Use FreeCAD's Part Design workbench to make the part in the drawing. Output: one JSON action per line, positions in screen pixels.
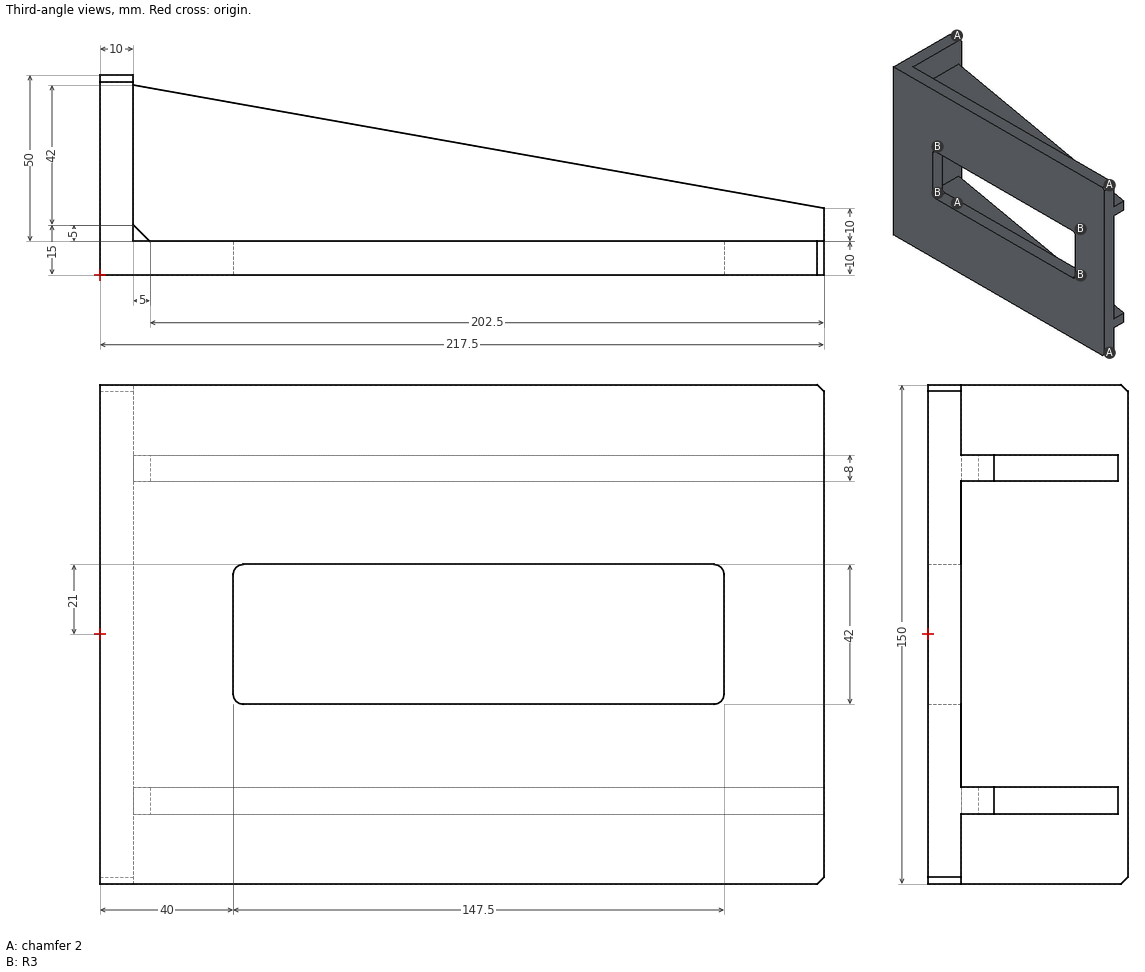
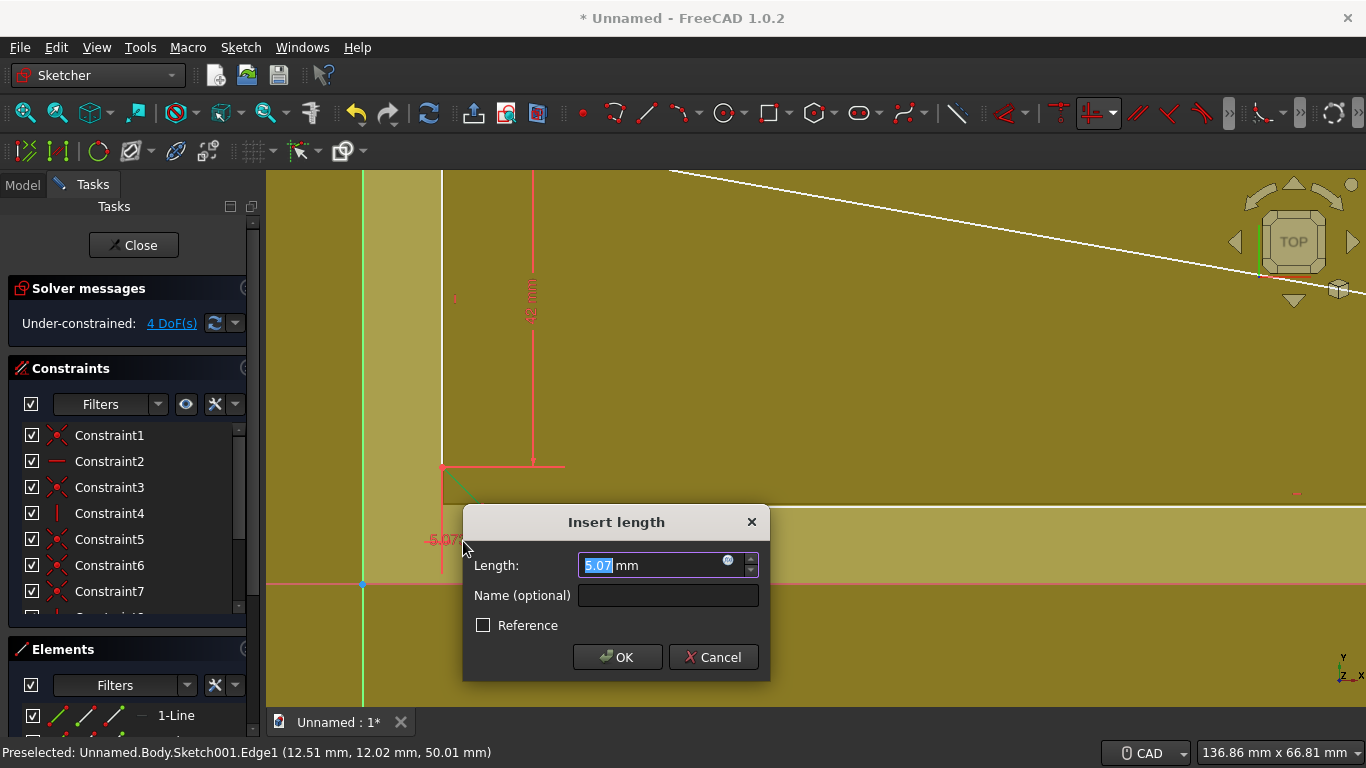
{"action": "type", "text": "5"}
{"action": "key", "text": "Return"}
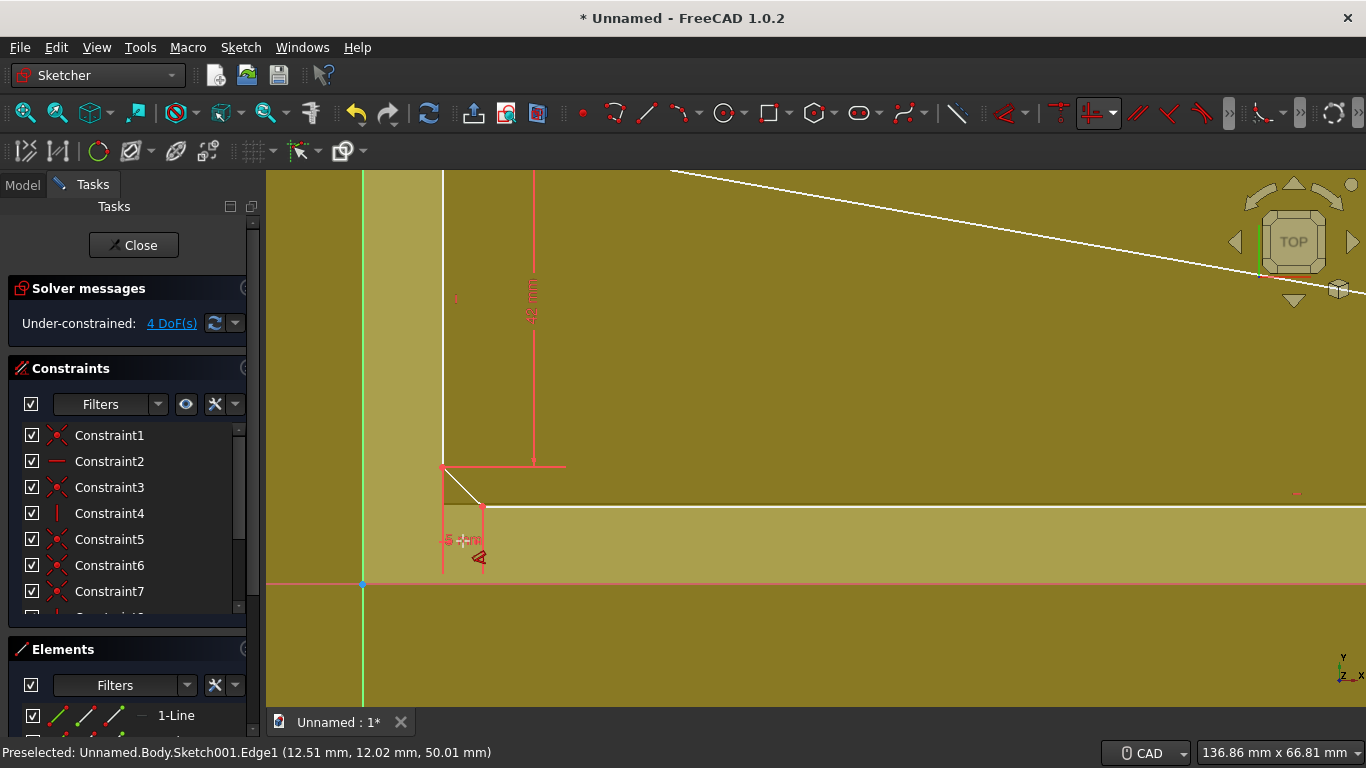
{"action": "left_click", "coordinate": [455, 479]}
{"action": "left_click", "coordinate": [409, 487]}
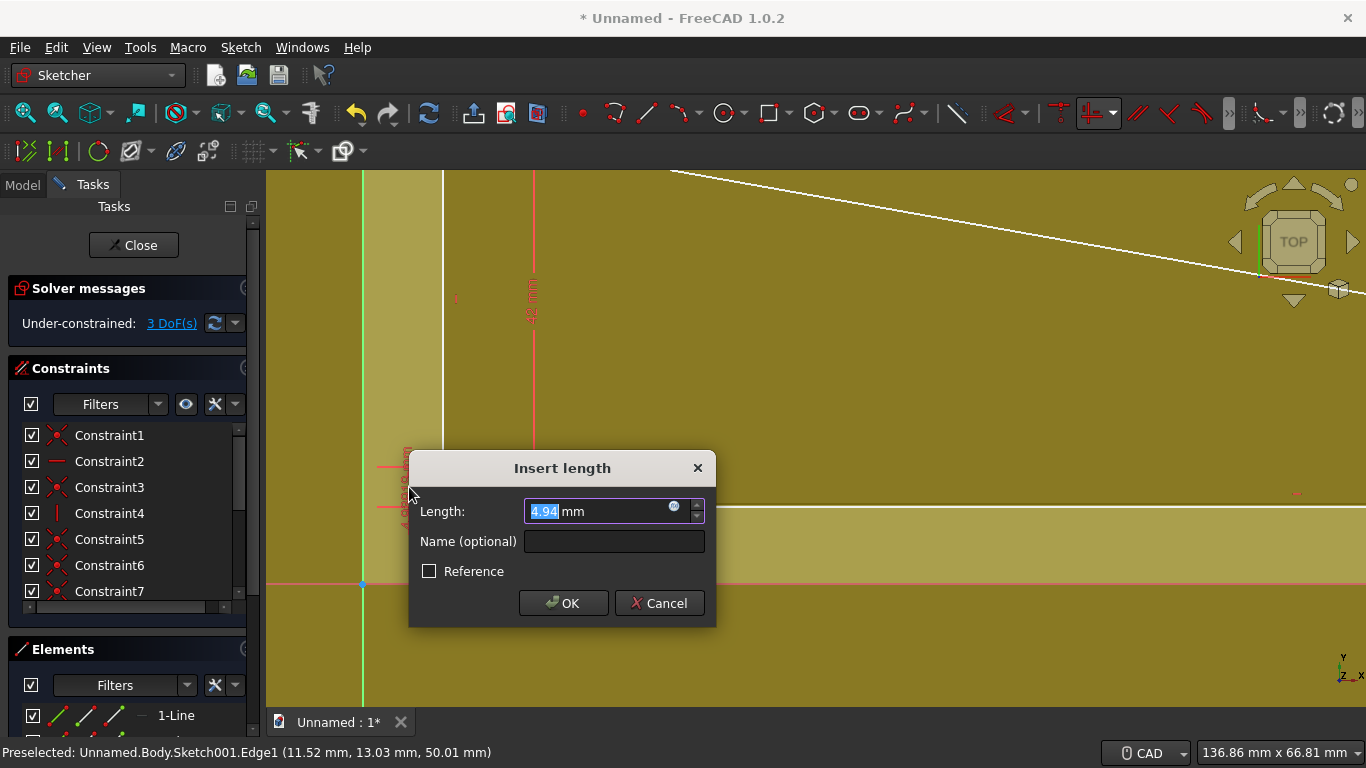
{"action": "type", "text": "5"}
{"action": "key", "text": "Return"}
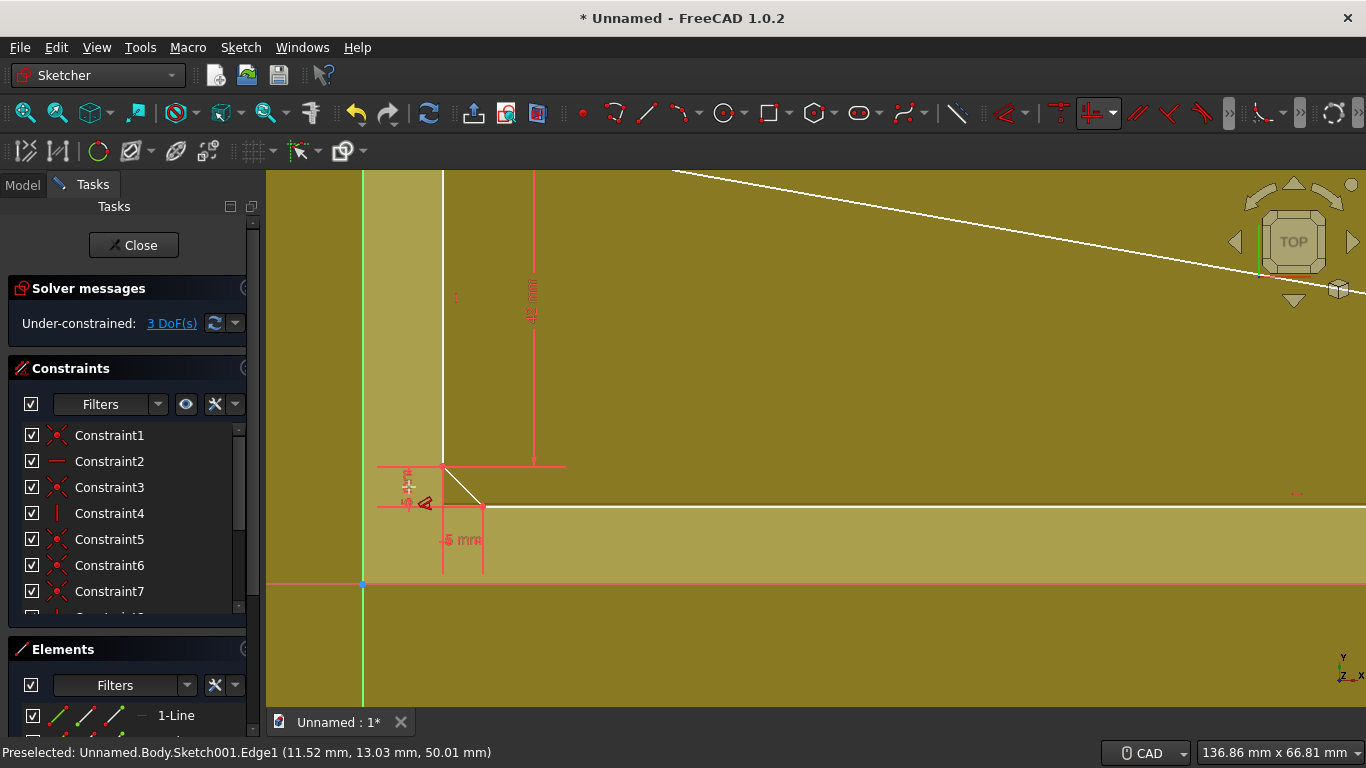
{"action": "left_click", "coordinate": [443, 467]}
{"action": "left_click", "coordinate": [403, 618]}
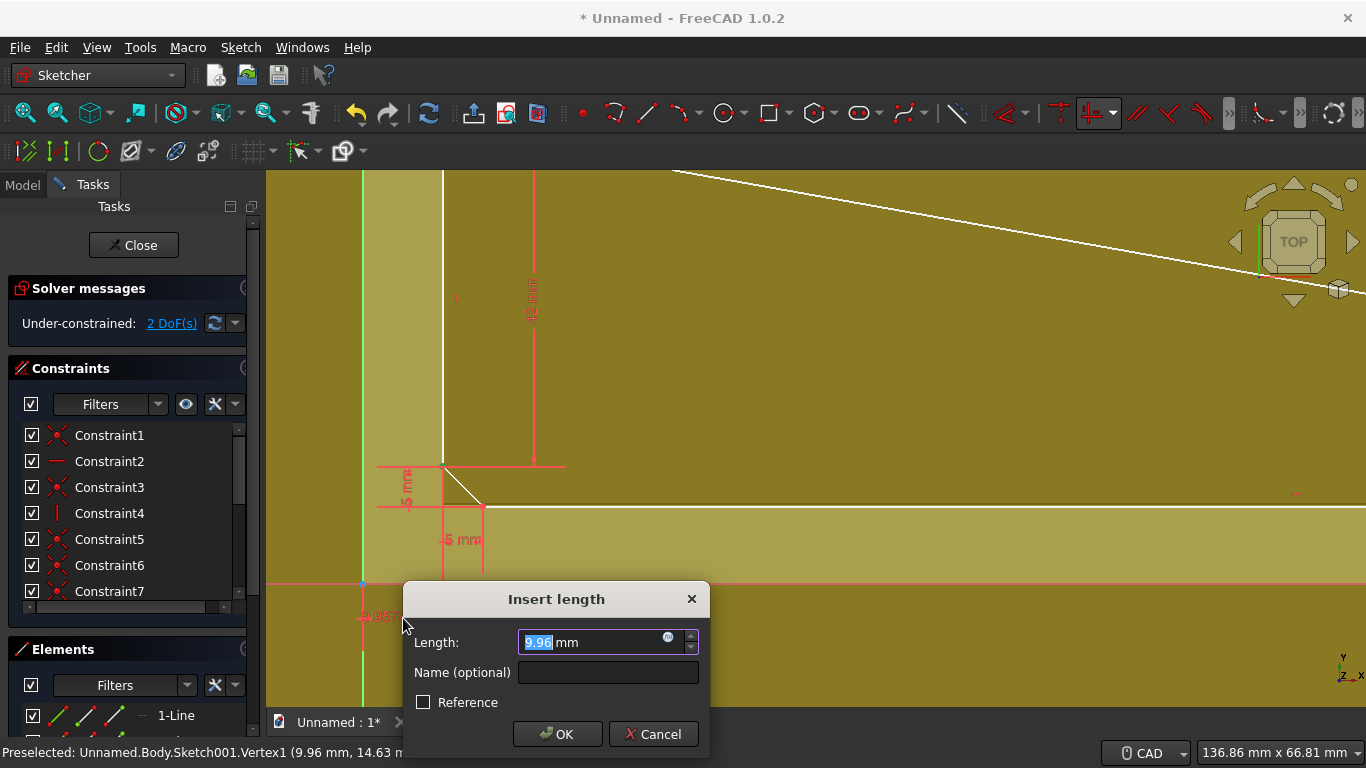
{"action": "type", "text": "10"}
{"action": "key", "text": "Return"}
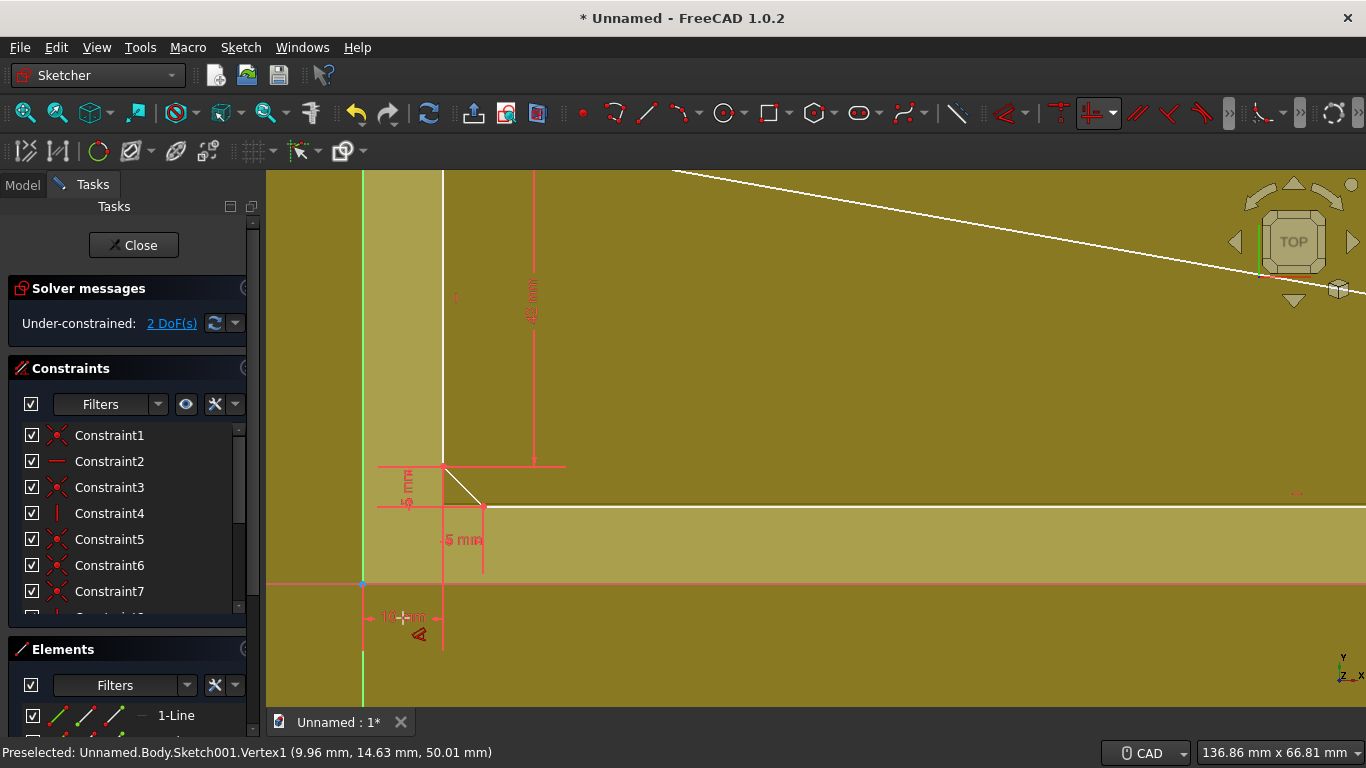
{"action": "left_click", "coordinate": [443, 467]}
{"action": "left_click", "coordinate": [329, 526]}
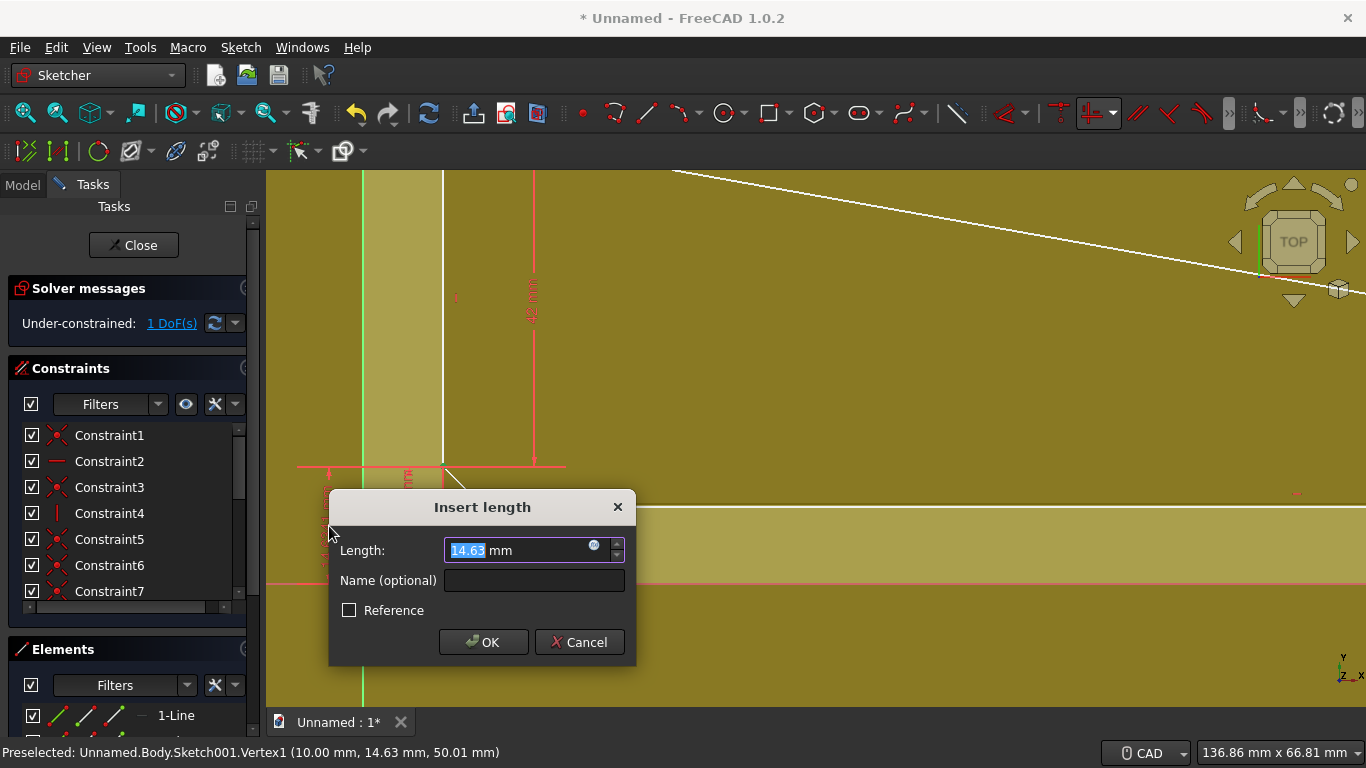
{"action": "type", "text": "15"}
{"action": "key", "text": "Return"}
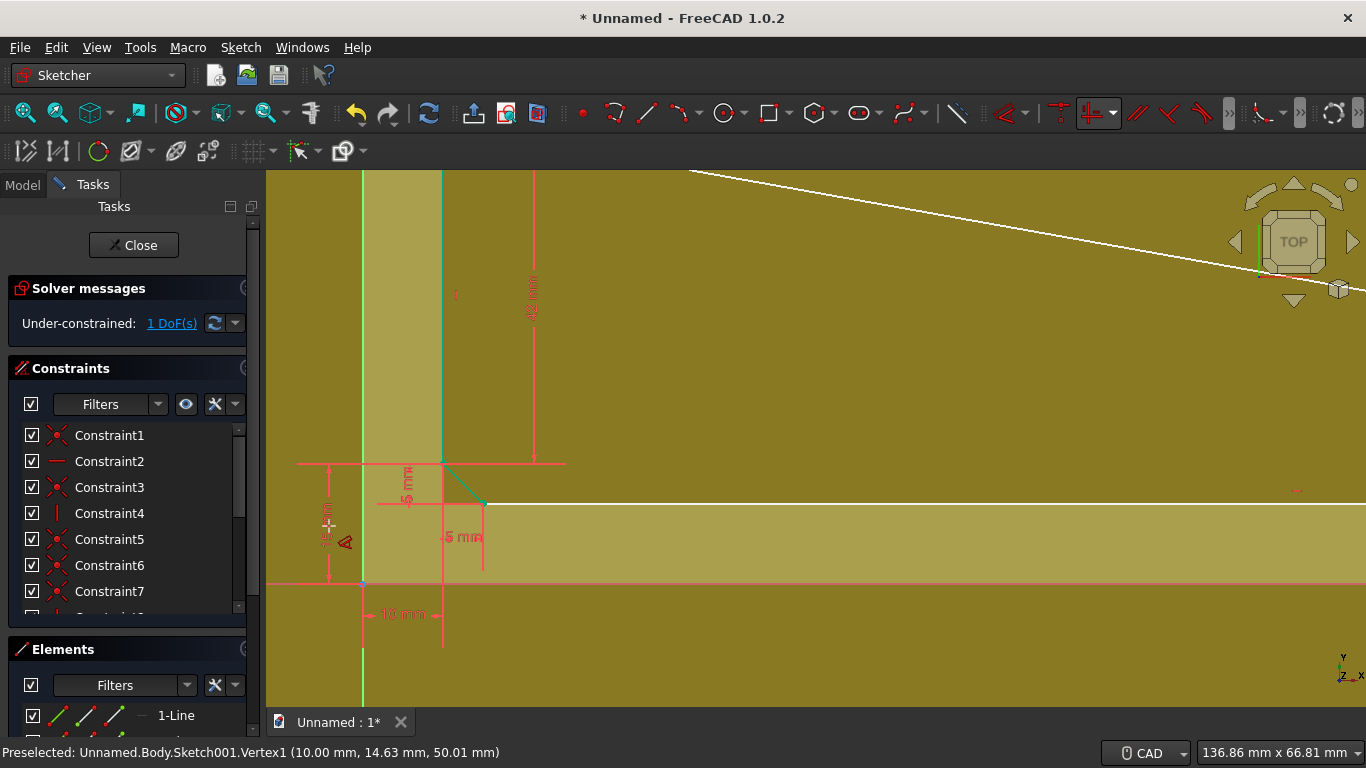
{"action": "left_click", "coordinate": [972, 504]}
{"action": "left_click", "coordinate": [842, 538]}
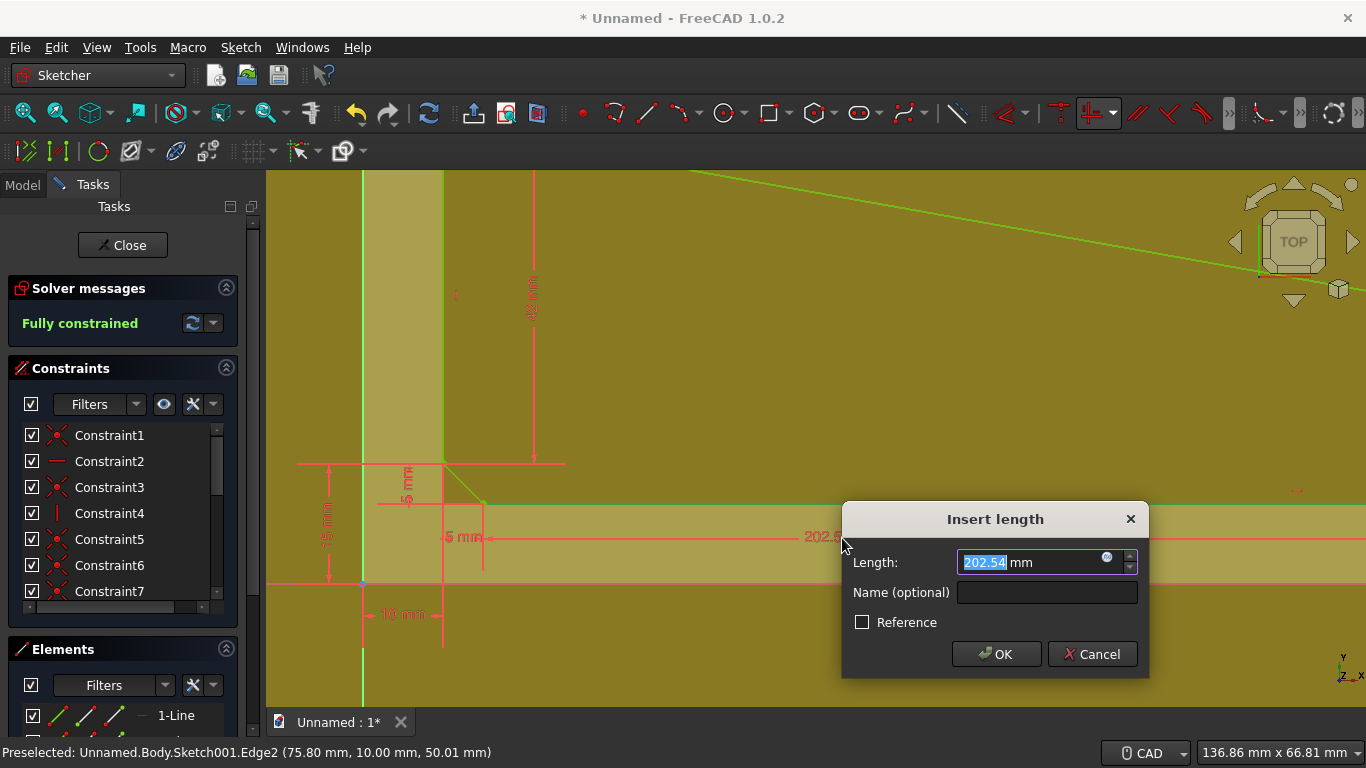
{"action": "type", "text": "202.5"}
{"action": "key", "text": "Return"}
{"action": "key", "text": "Escape"}